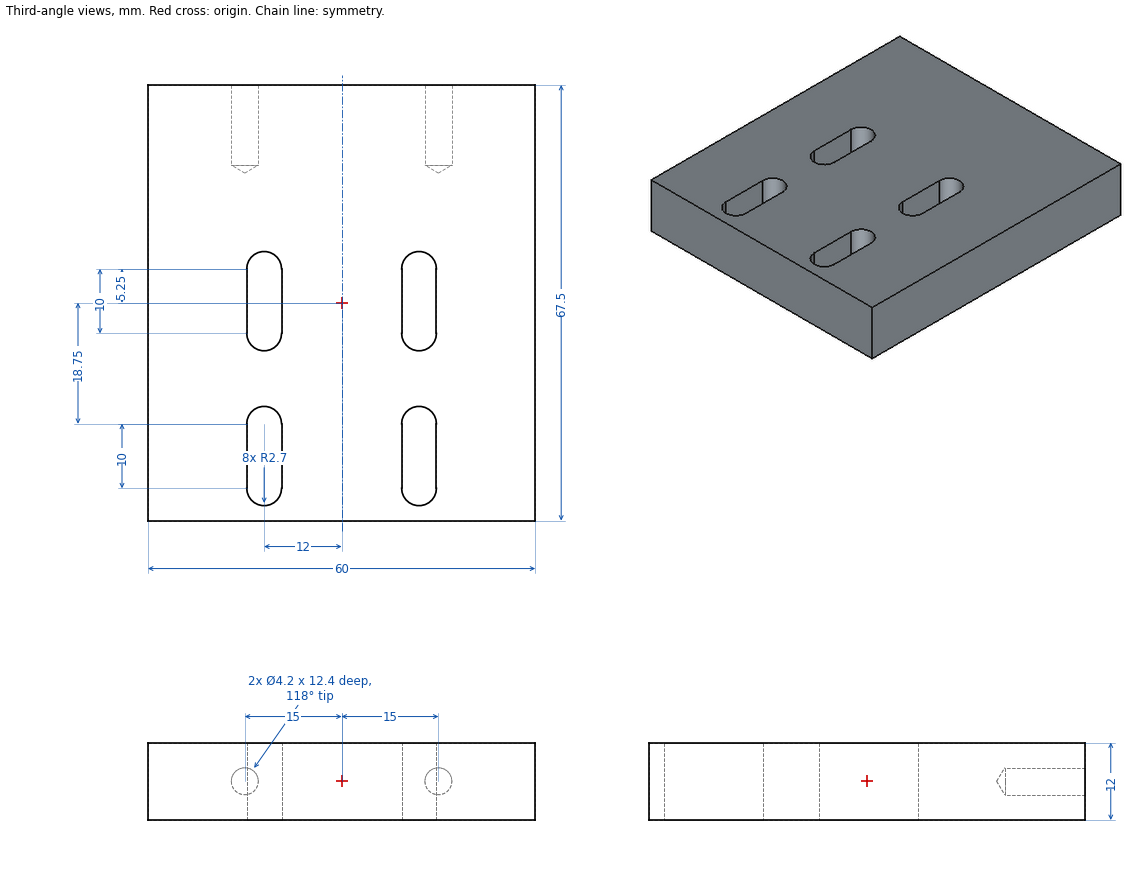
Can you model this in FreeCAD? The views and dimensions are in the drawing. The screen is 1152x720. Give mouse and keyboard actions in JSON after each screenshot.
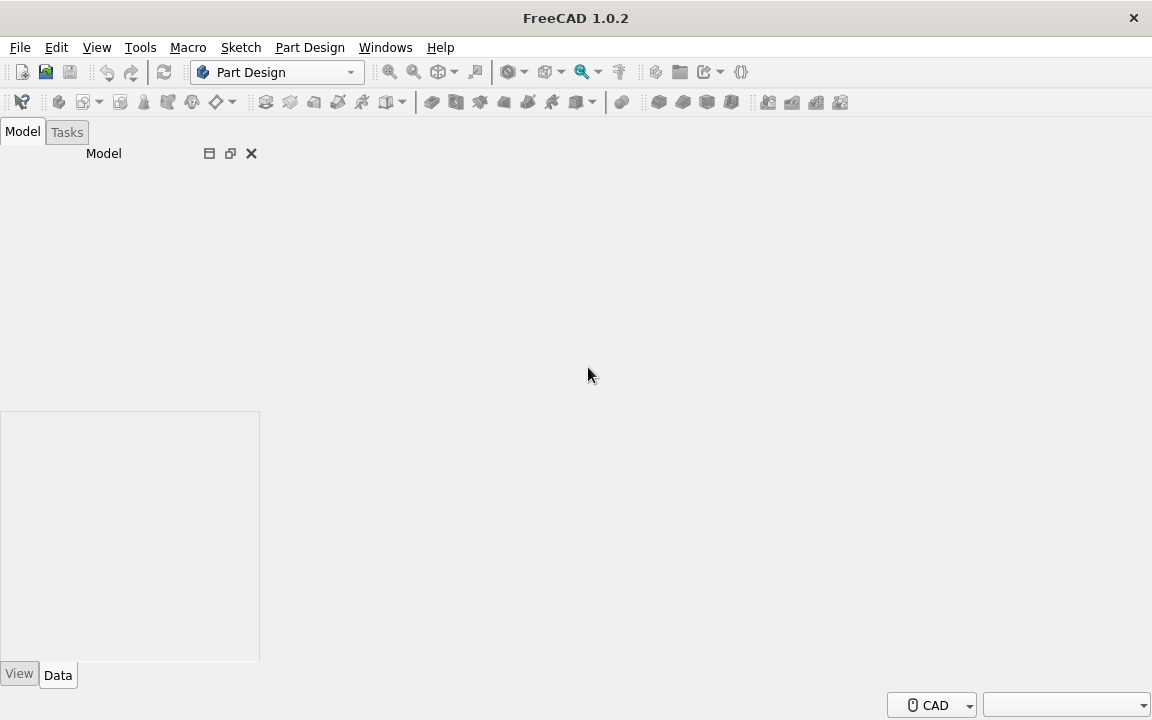
{"action": "key", "text": "ctrl+n"}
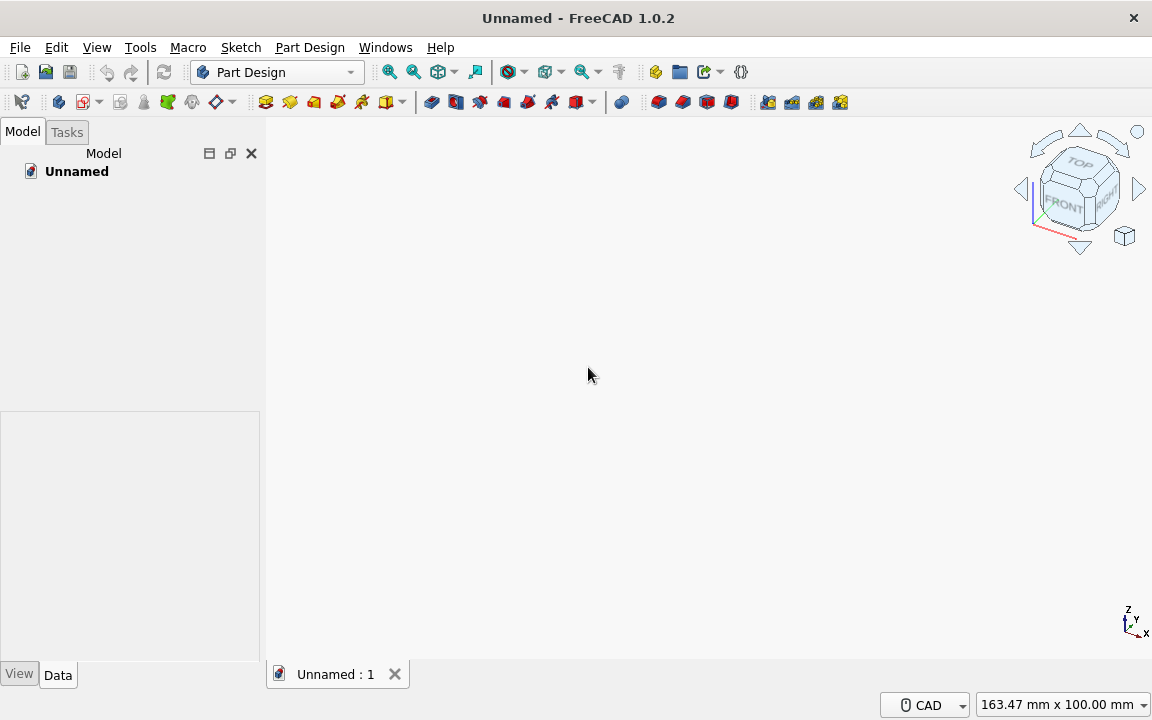
{"action": "left_click", "coordinate": [84, 102]}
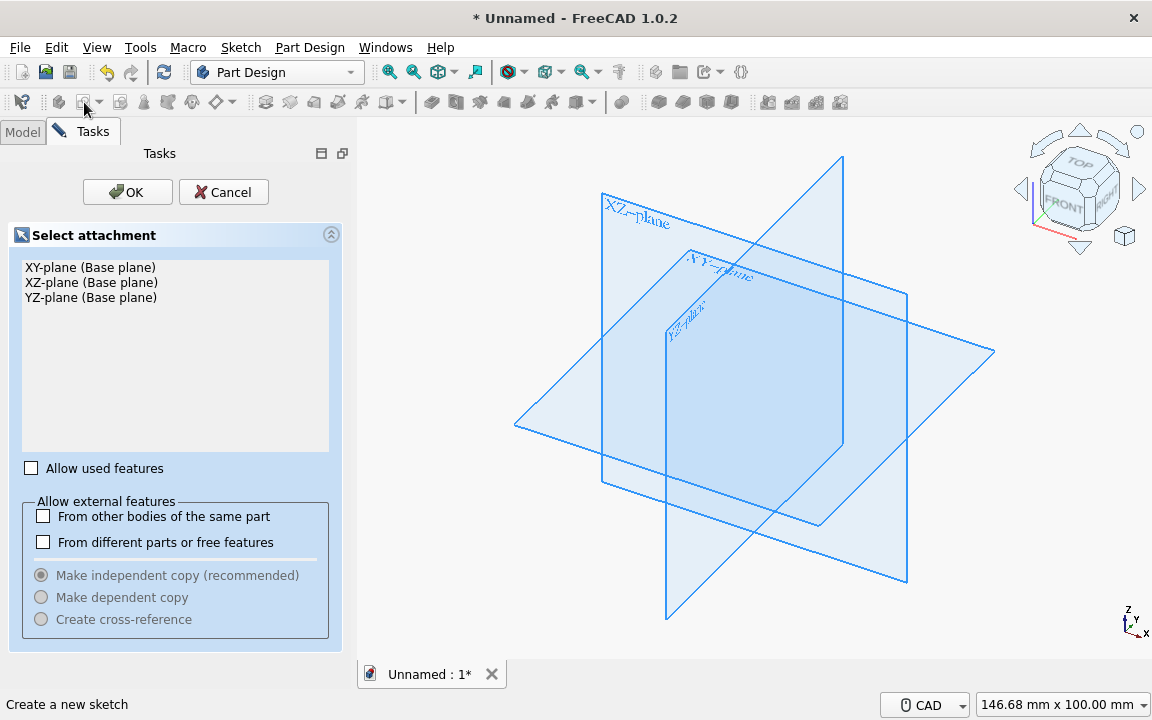
{"action": "left_click", "coordinate": [82, 268]}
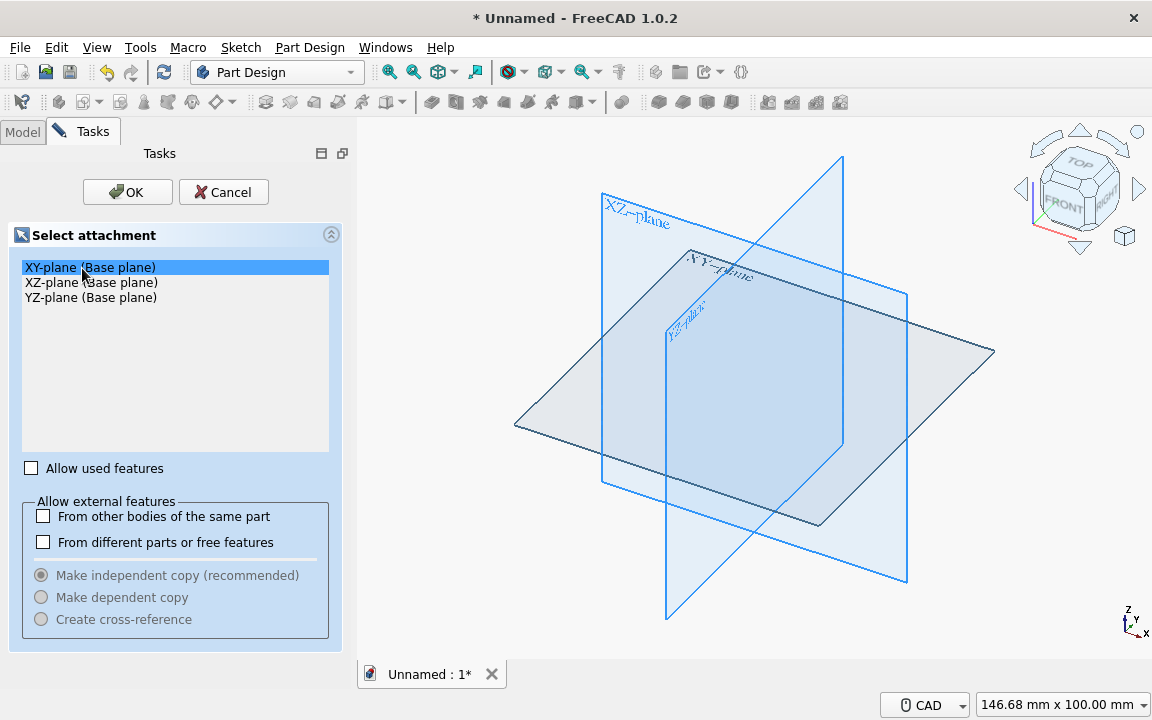
{"action": "left_click", "coordinate": [128, 192]}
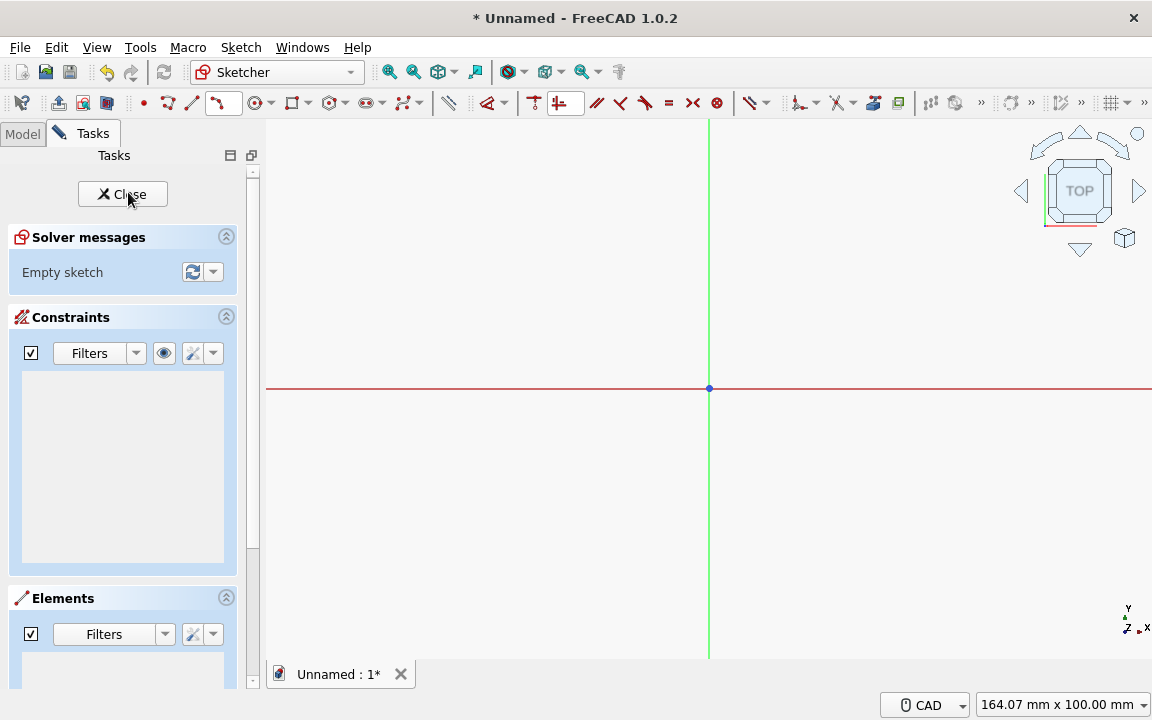
{"action": "key", "text": "g v"}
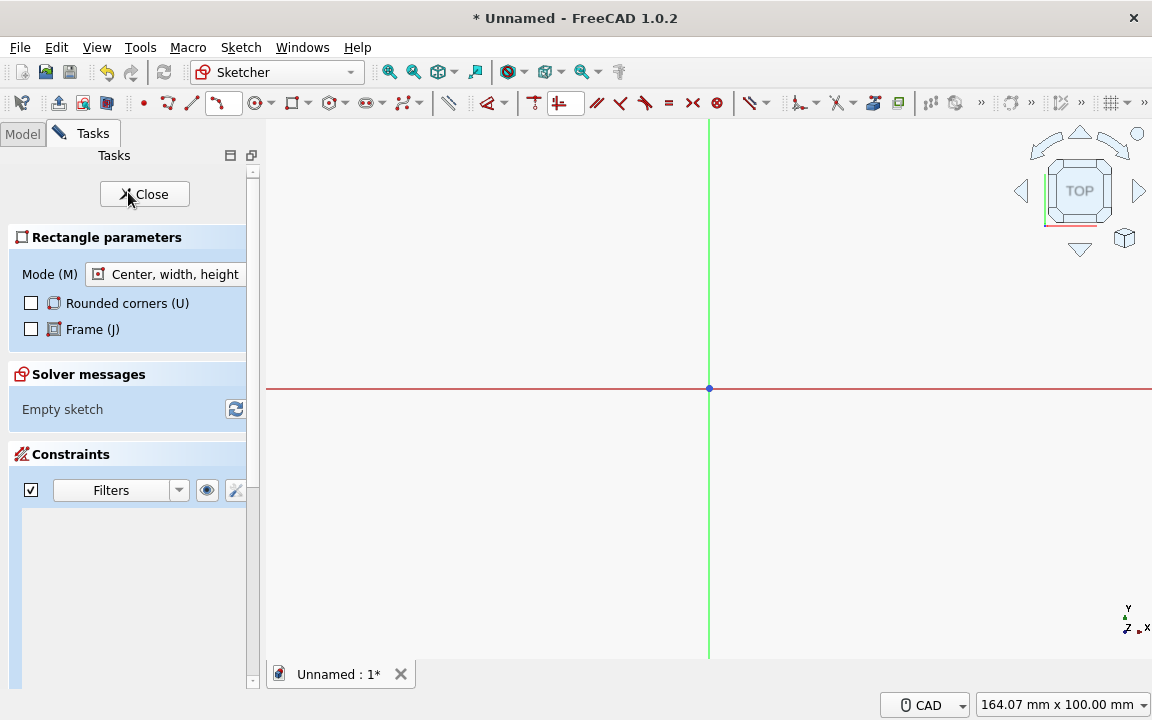
{"action": "left_click", "coordinate": [709, 389]}
{"action": "mouse_move", "coordinate": [871, 207]}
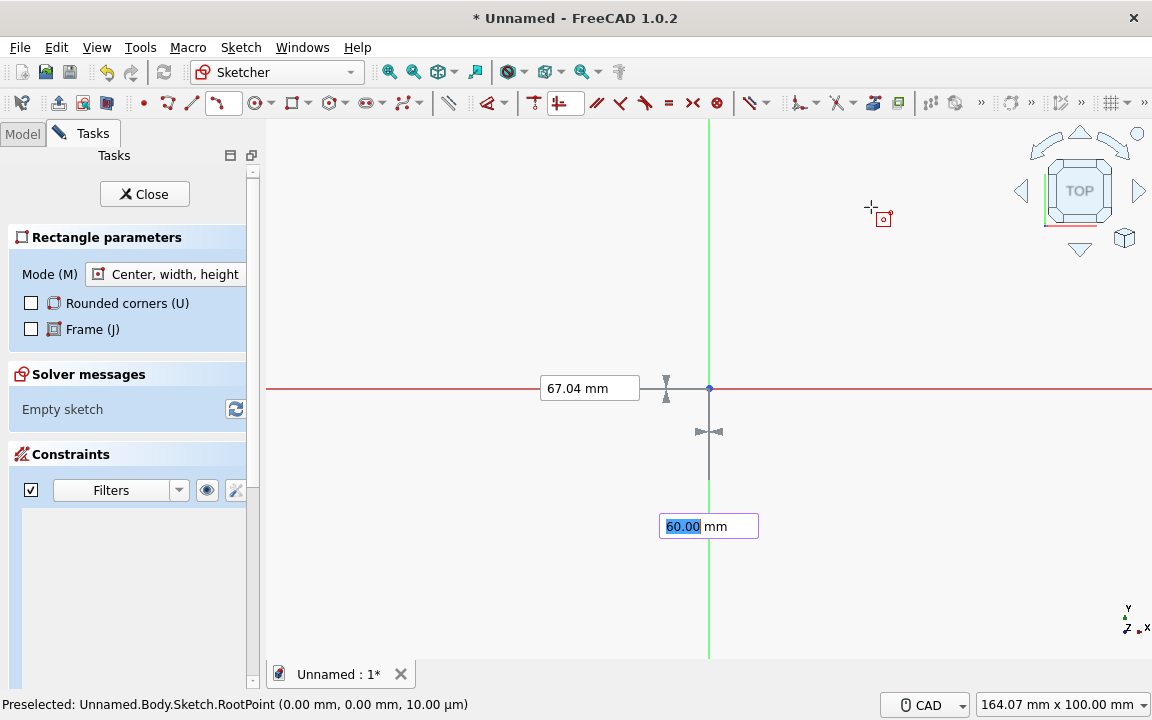
{"action": "type", "text": "60"}
{"action": "key", "text": "Tab"}
{"action": "type", "text": "67.5"}
{"action": "key", "text": "Return"}
{"action": "key", "text": "Escape"}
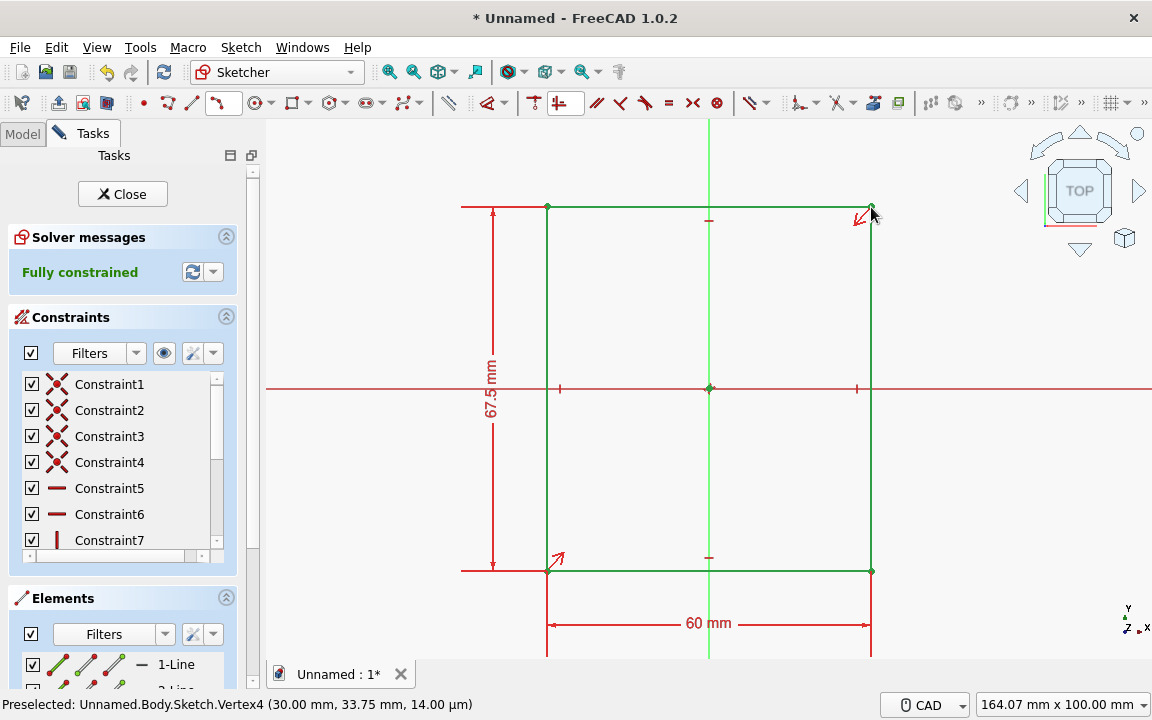
{"action": "left_click", "coordinate": [123, 194]}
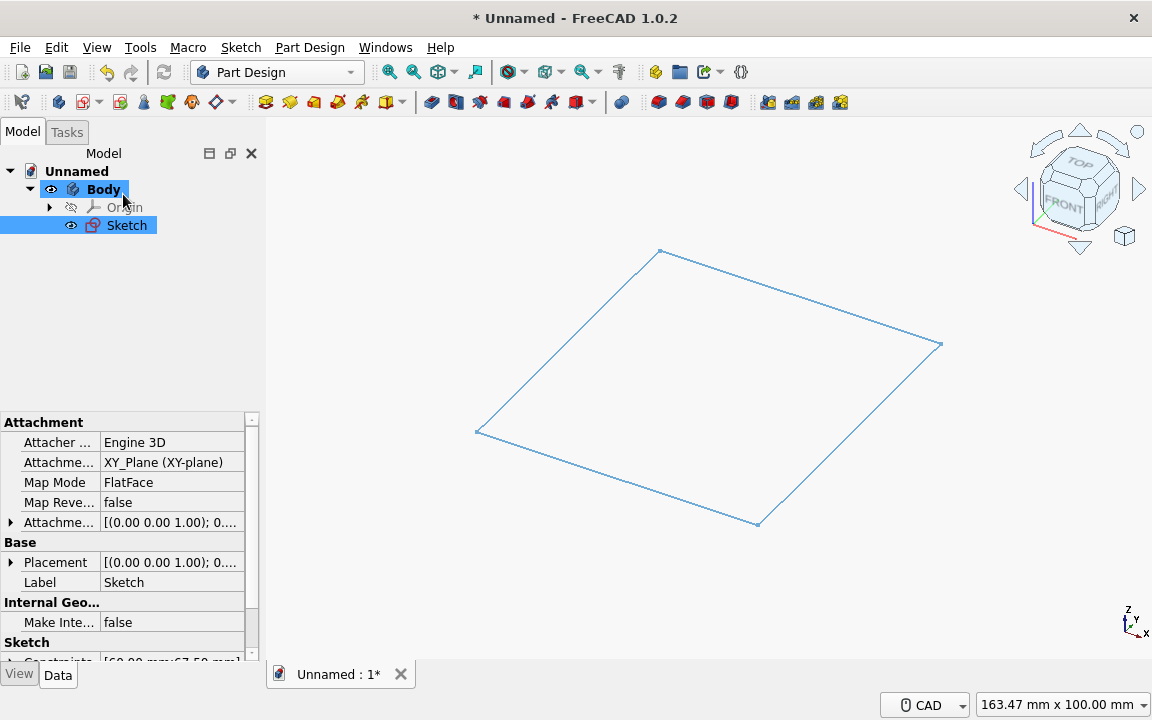
{"action": "left_click", "coordinate": [266, 102]}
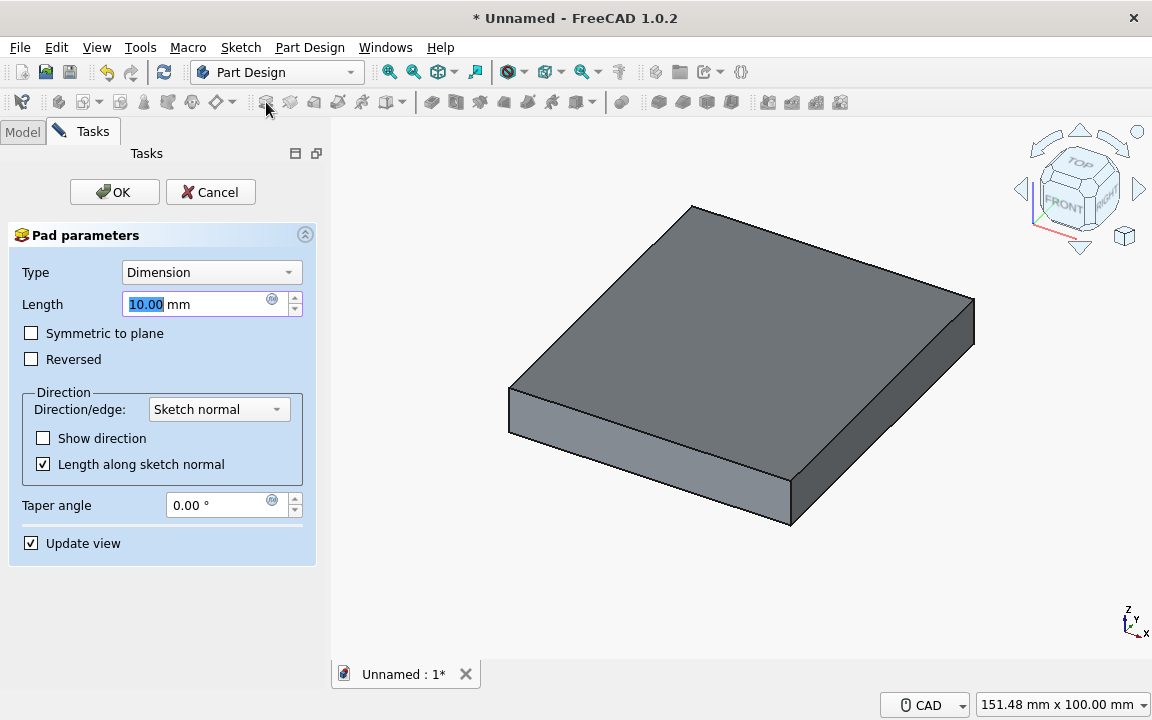
{"action": "type", "text": "12"}
{"action": "key", "text": "Tab"}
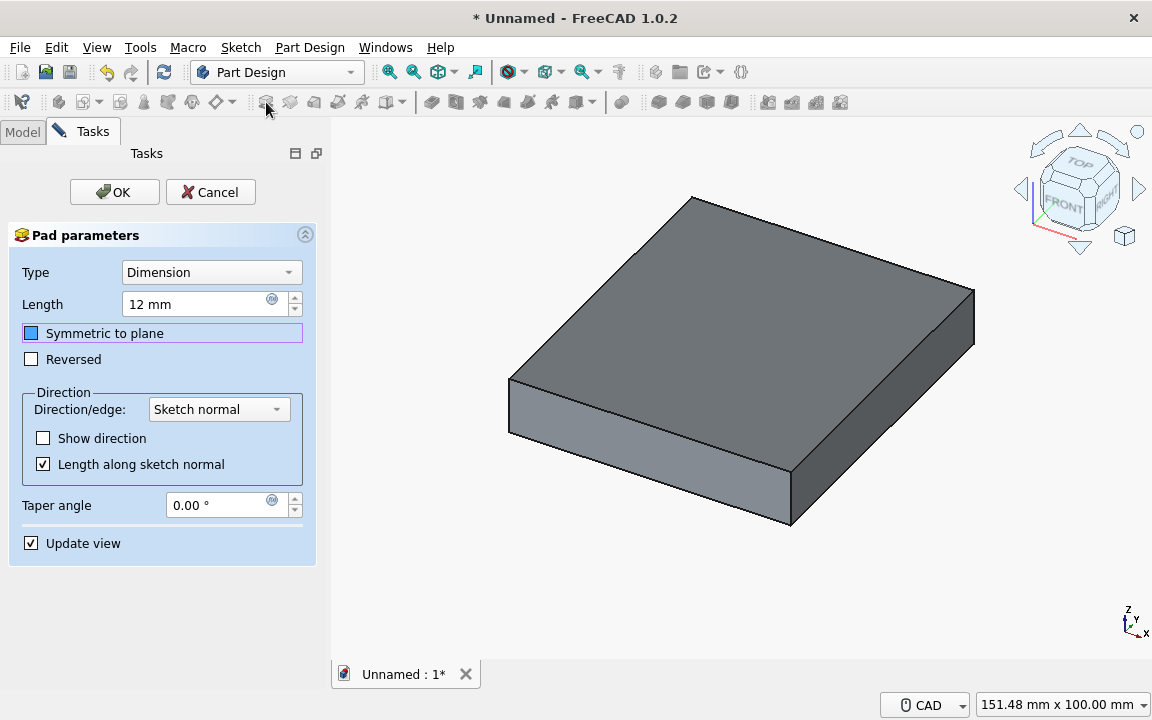
{"action": "left_click", "coordinate": [30, 333]}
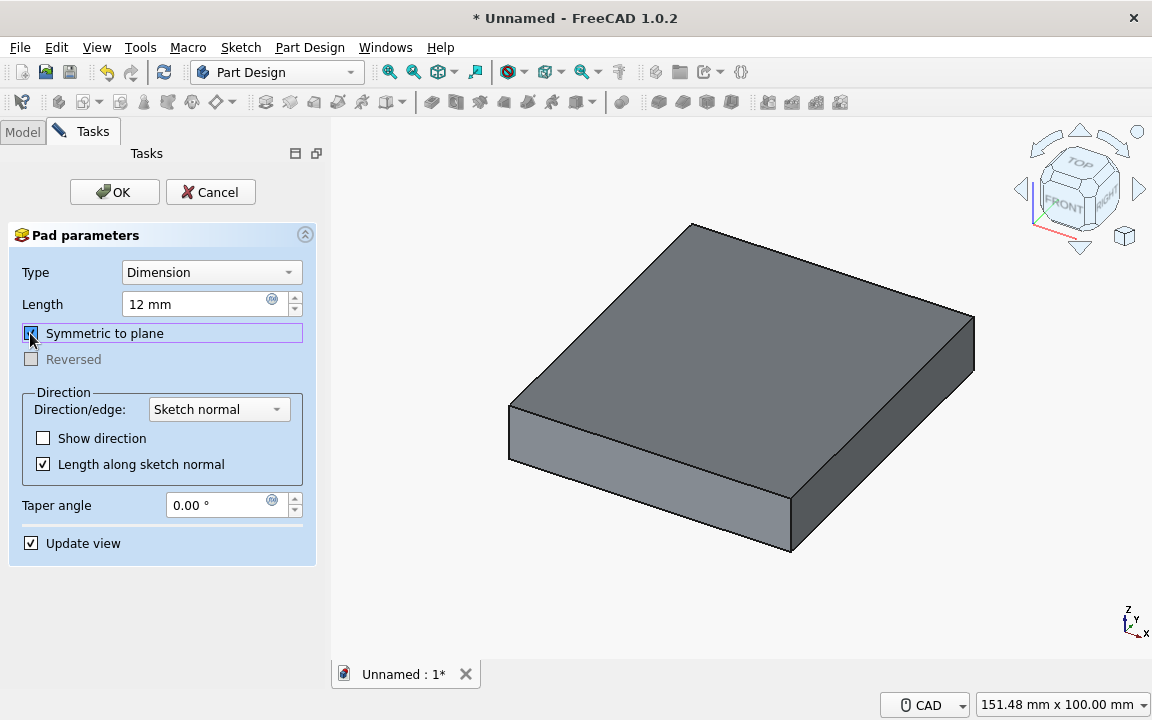
{"action": "left_click", "coordinate": [115, 192]}